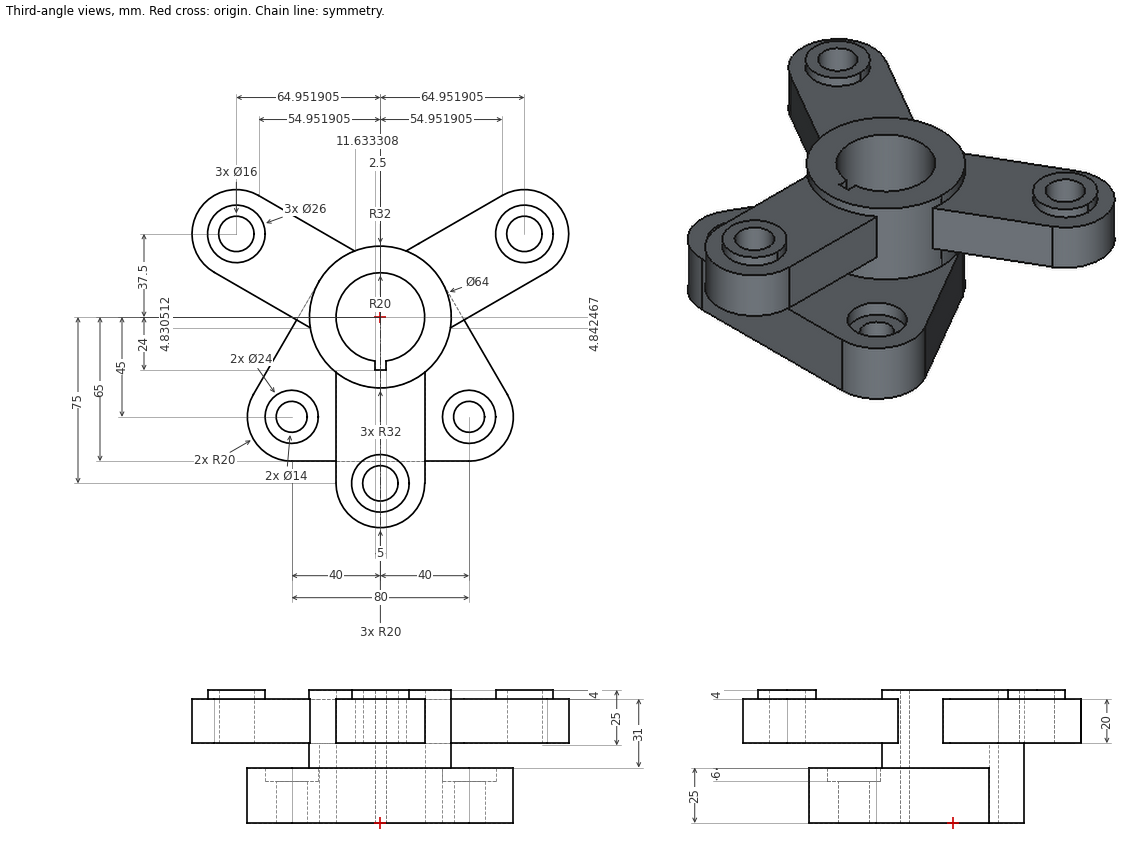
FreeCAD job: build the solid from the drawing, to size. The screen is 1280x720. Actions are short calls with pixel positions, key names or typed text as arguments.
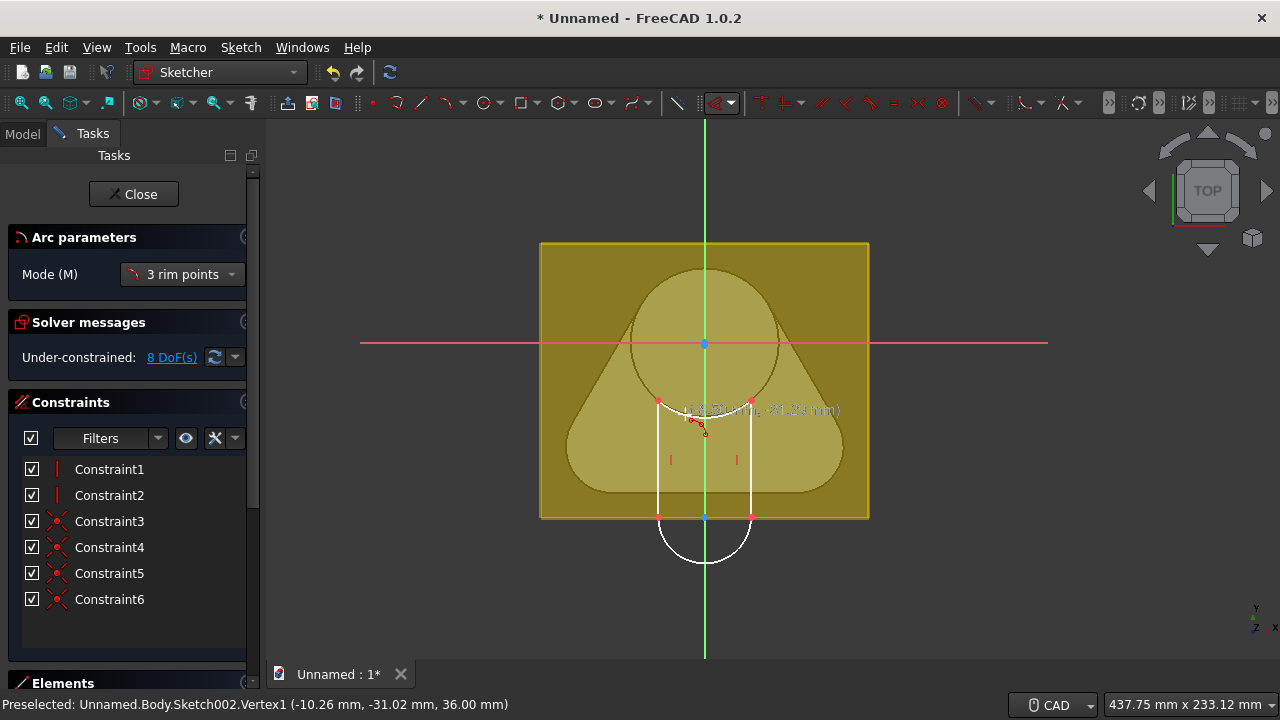
key(g)
key(l)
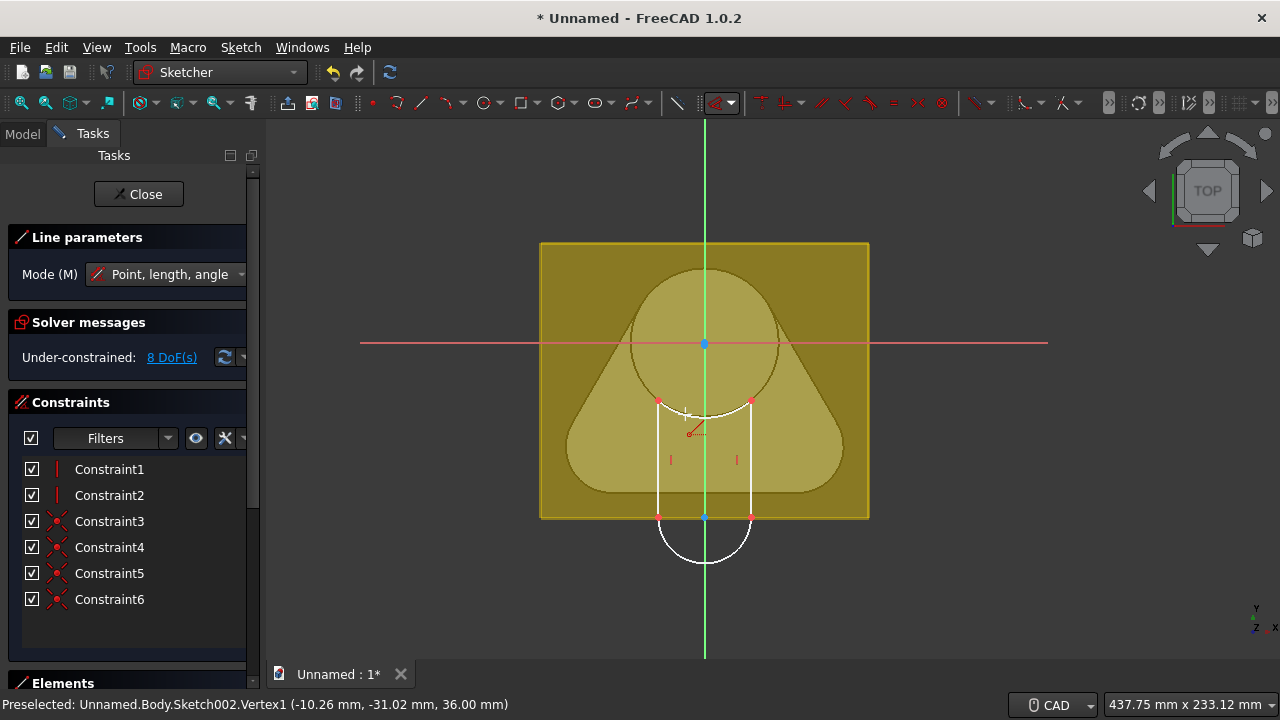
click(678, 273)
click(577, 216)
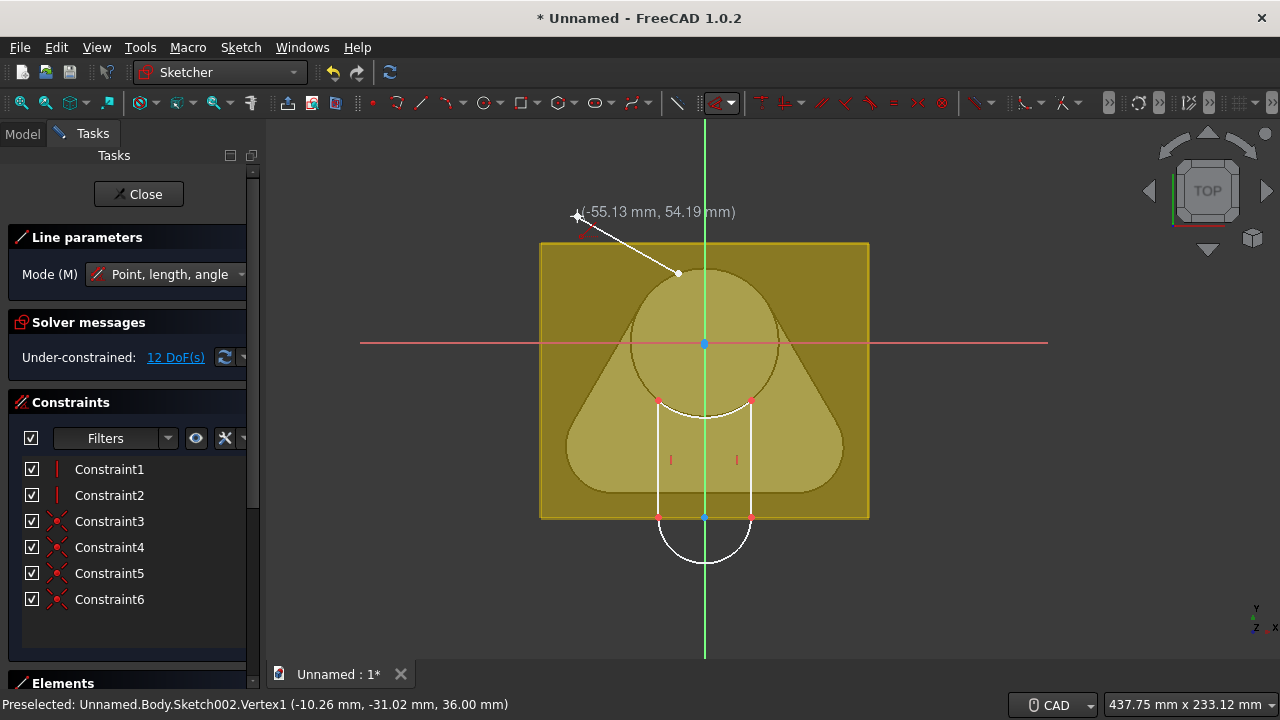
click(531, 296)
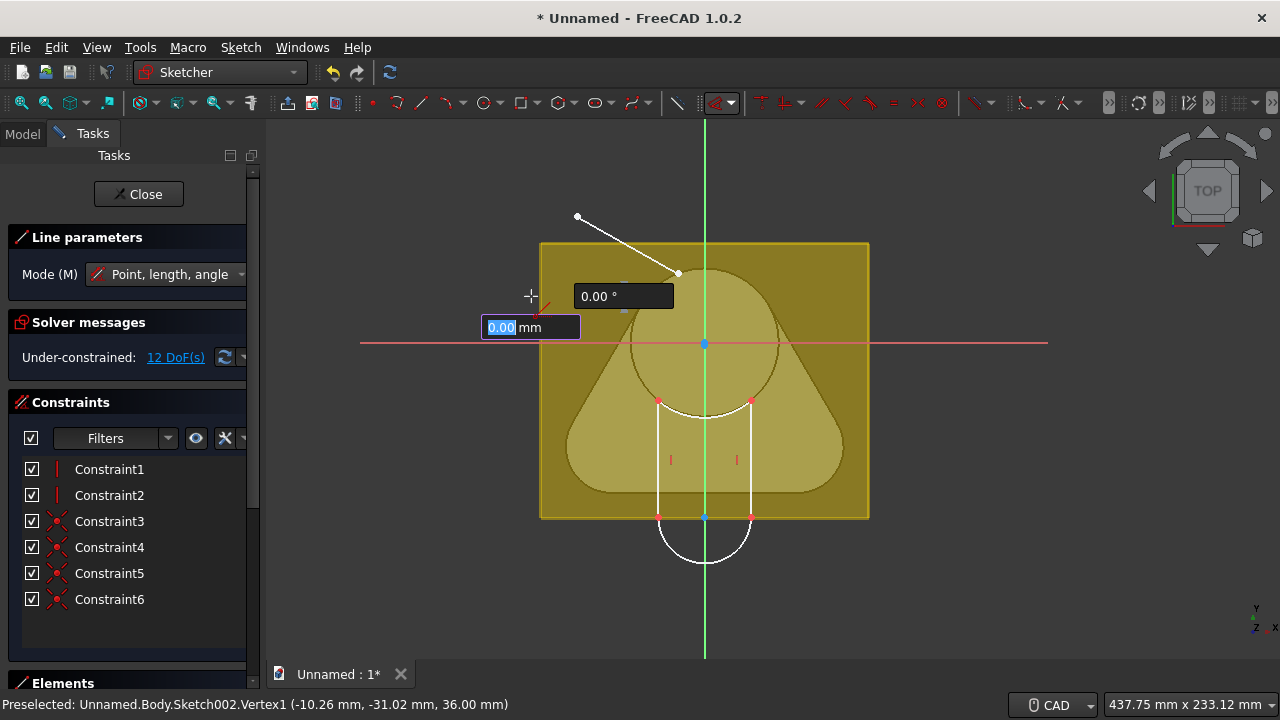
scroll(631, 354, up, 2)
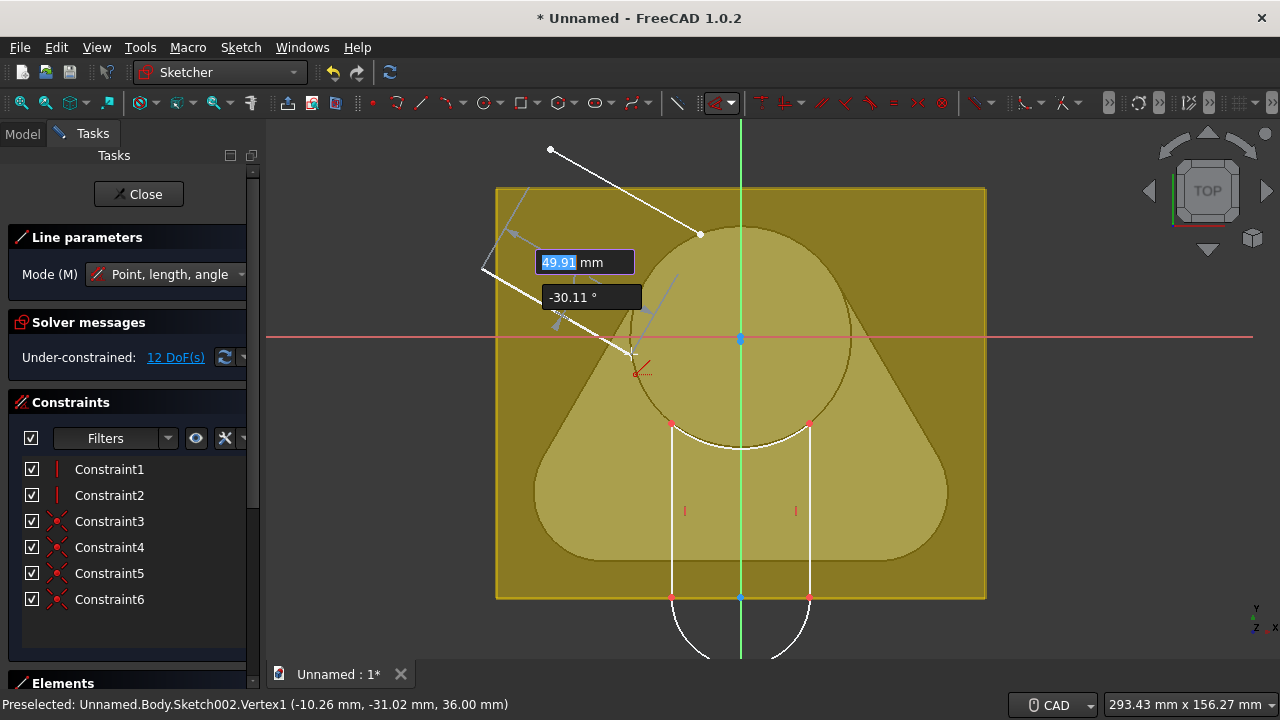
click(631, 353)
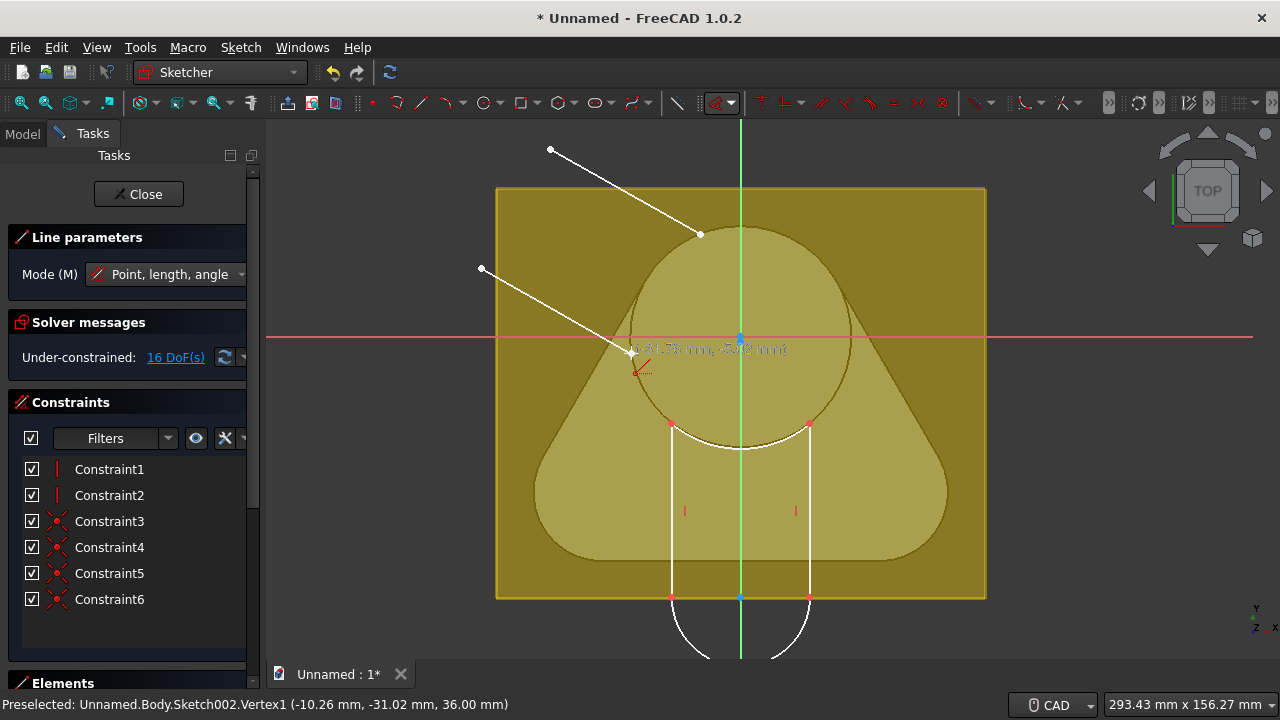
key(g)
key(3)
key(a)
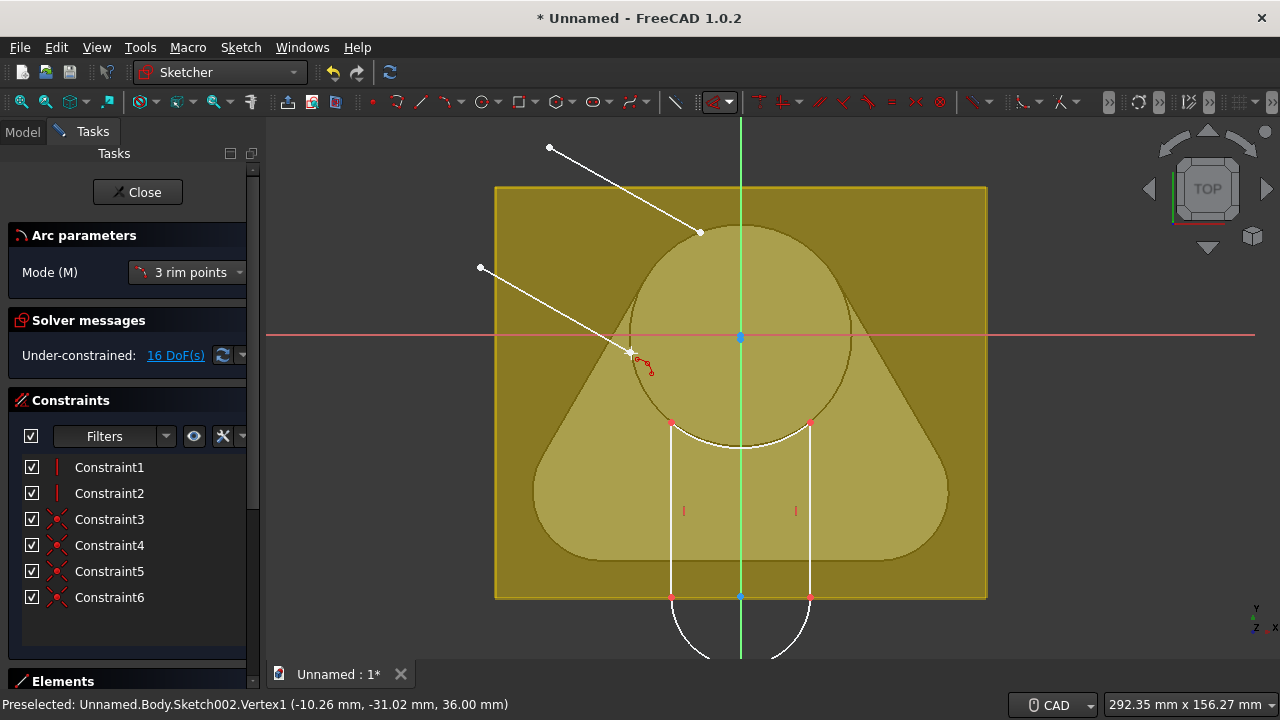
click(549, 148)
click(481, 267)
click(455, 171)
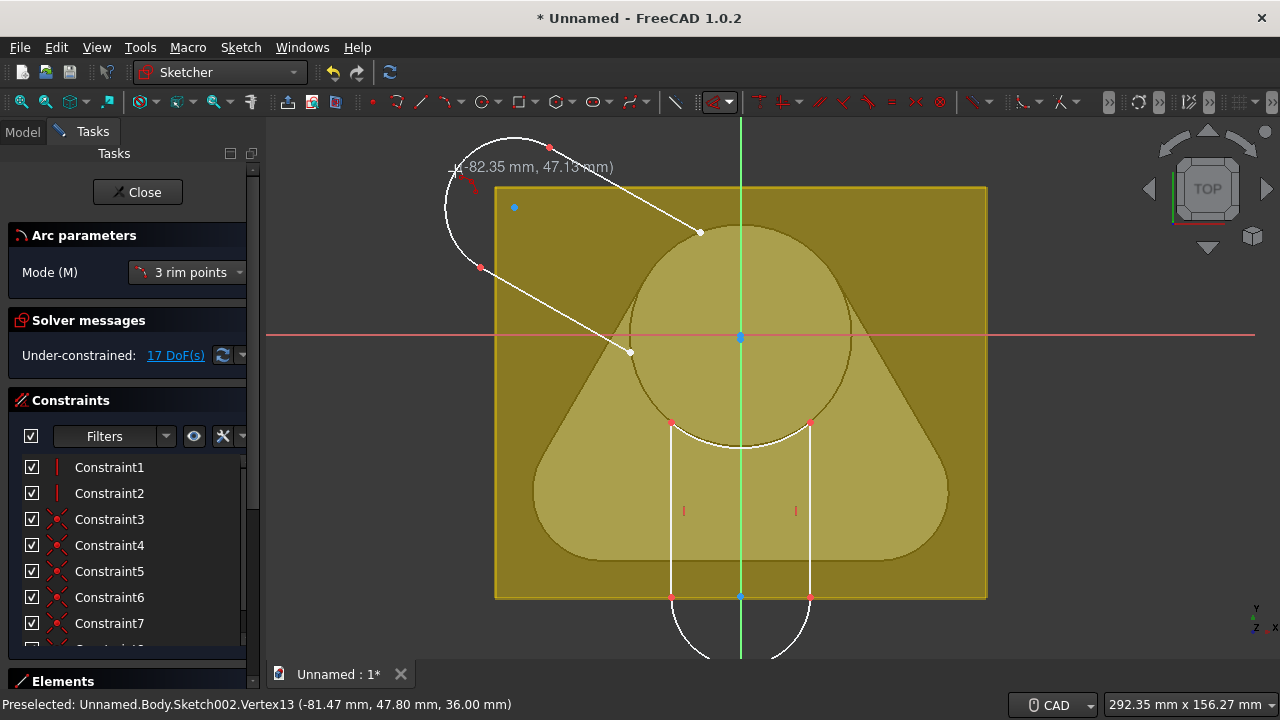
click(630, 353)
click(701, 233)
click(645, 280)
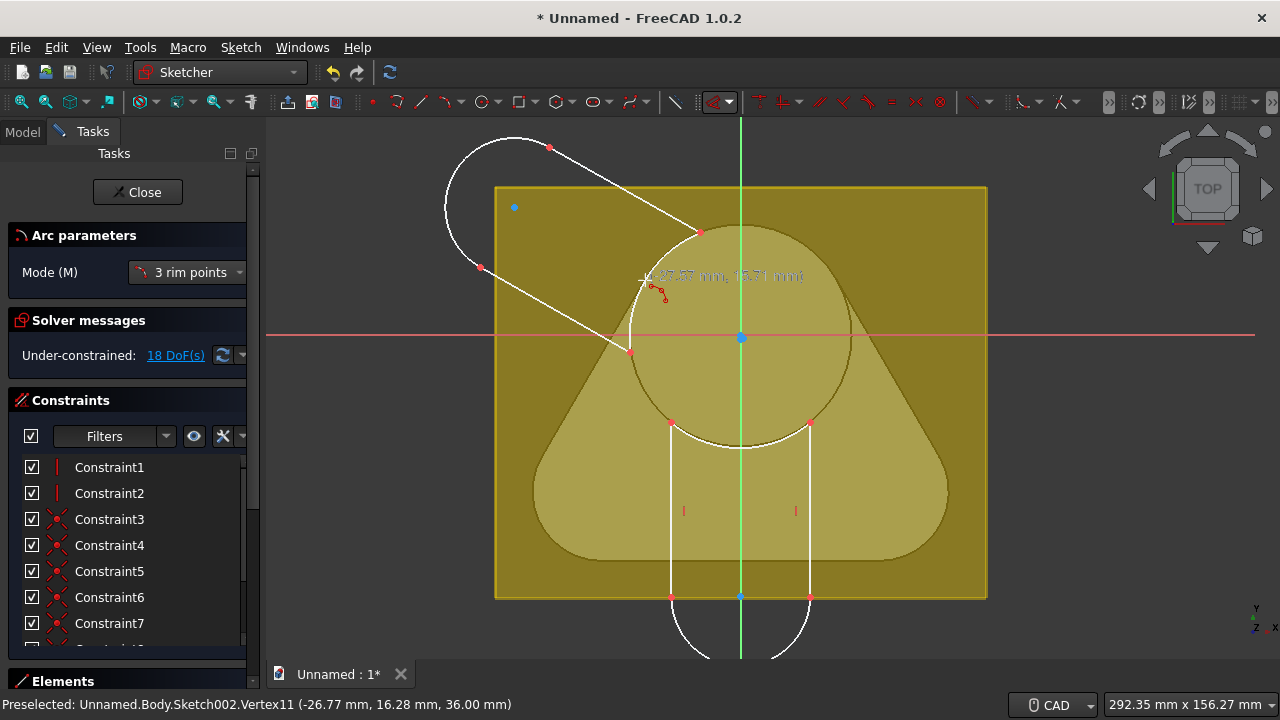
key(g)
key(l)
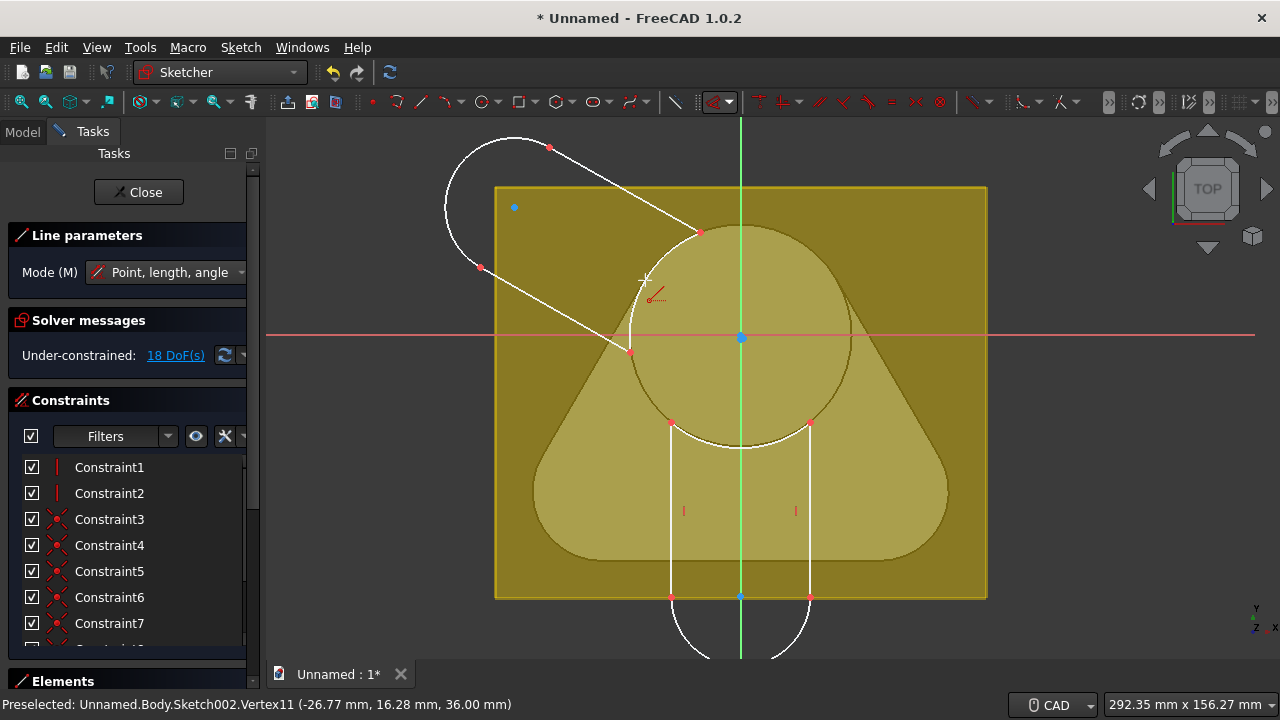
click(931, 145)
click(781, 232)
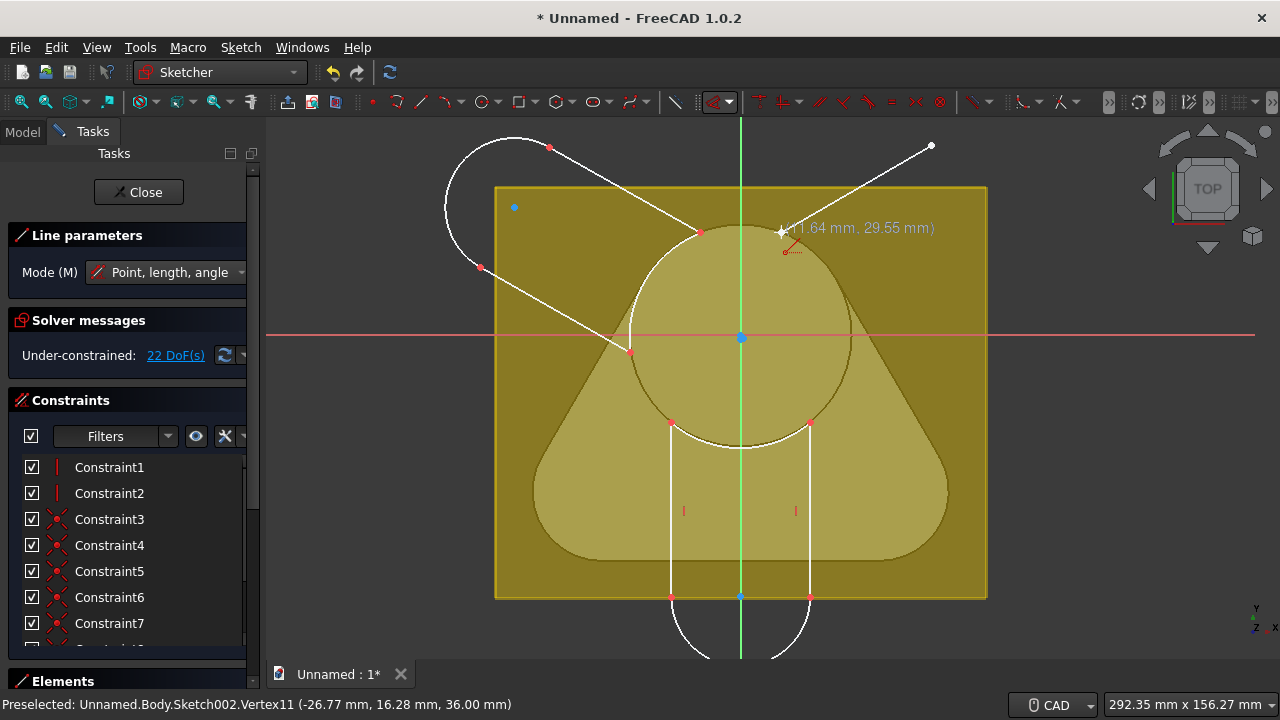
click(850, 352)
click(1001, 265)